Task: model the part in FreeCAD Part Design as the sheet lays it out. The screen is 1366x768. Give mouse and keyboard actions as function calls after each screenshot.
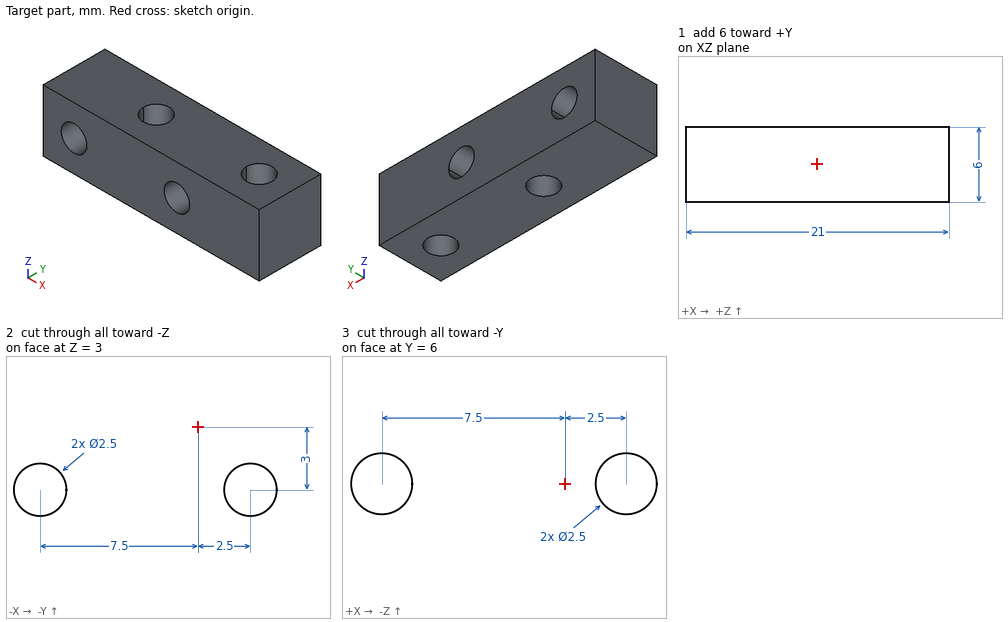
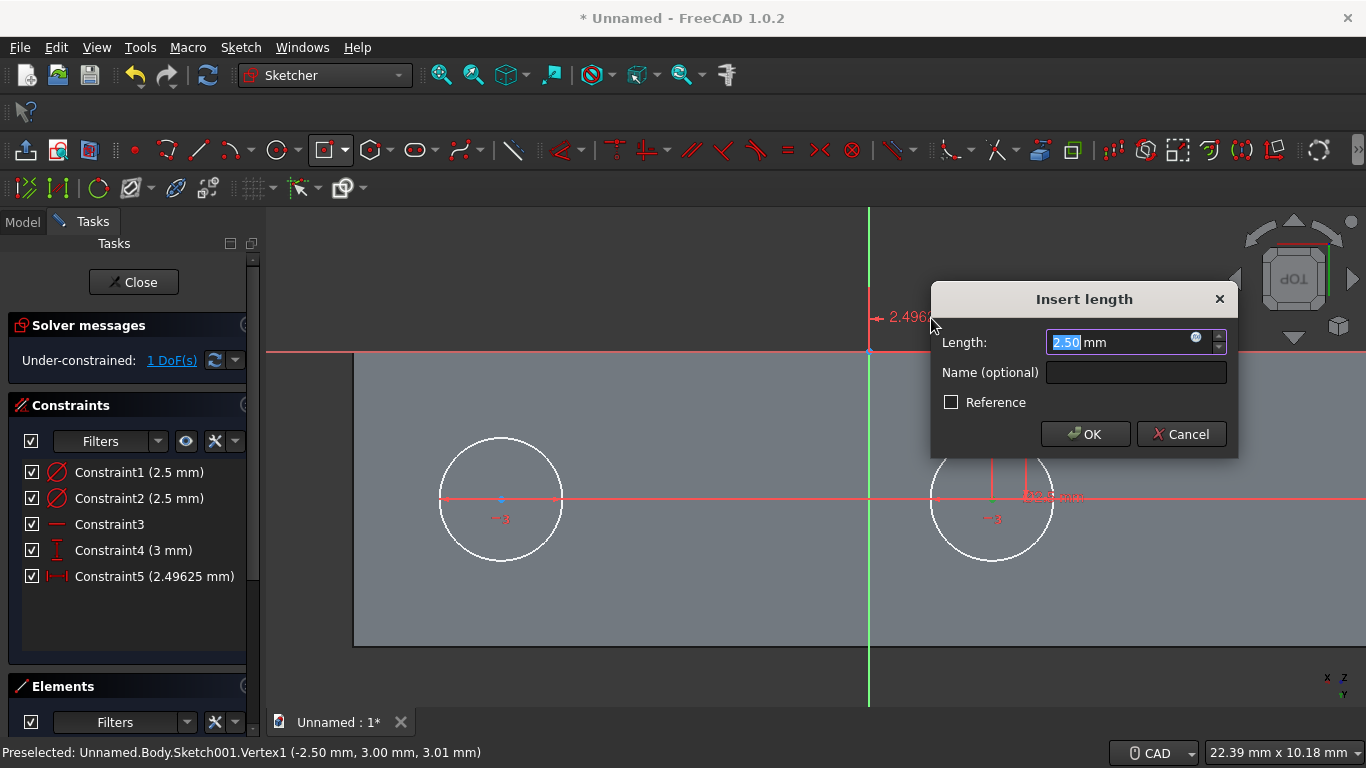
text(2.5)
key(Return)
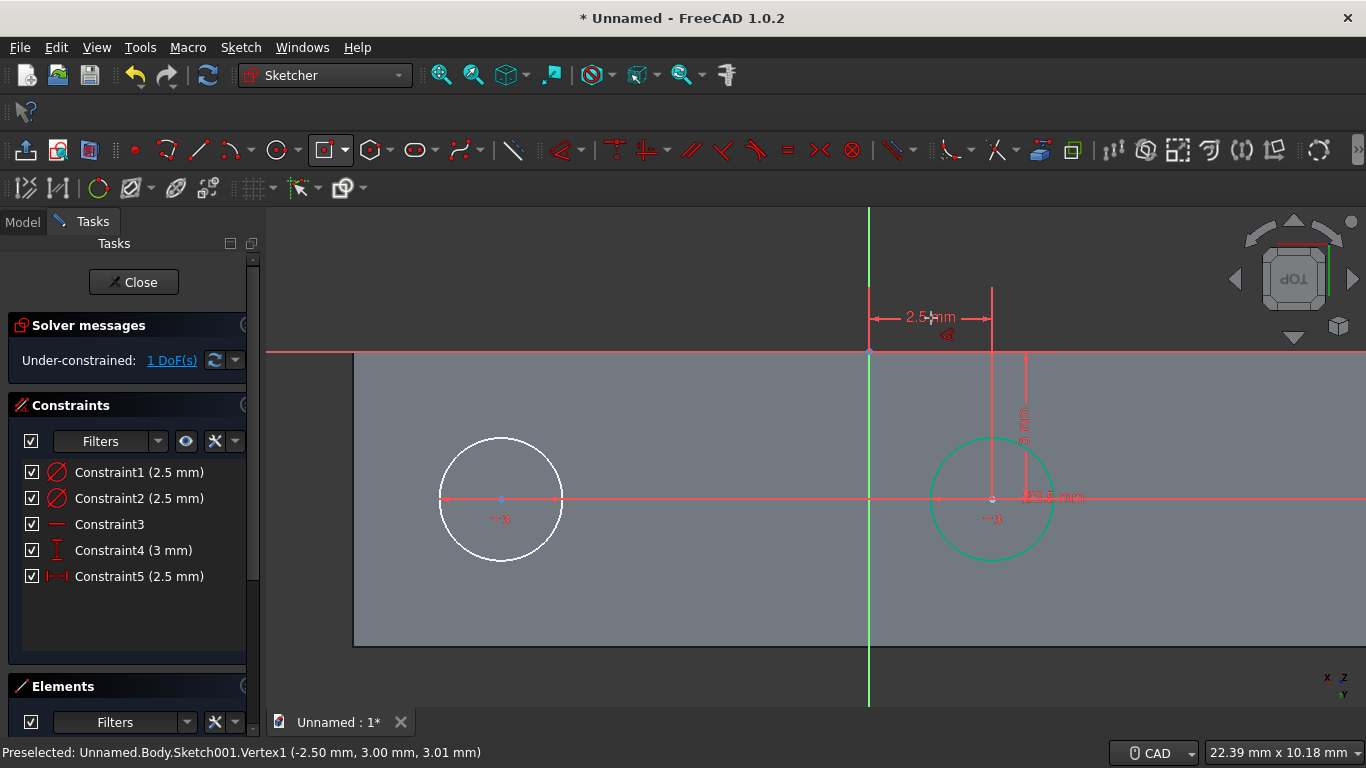
click(501, 499)
click(685, 318)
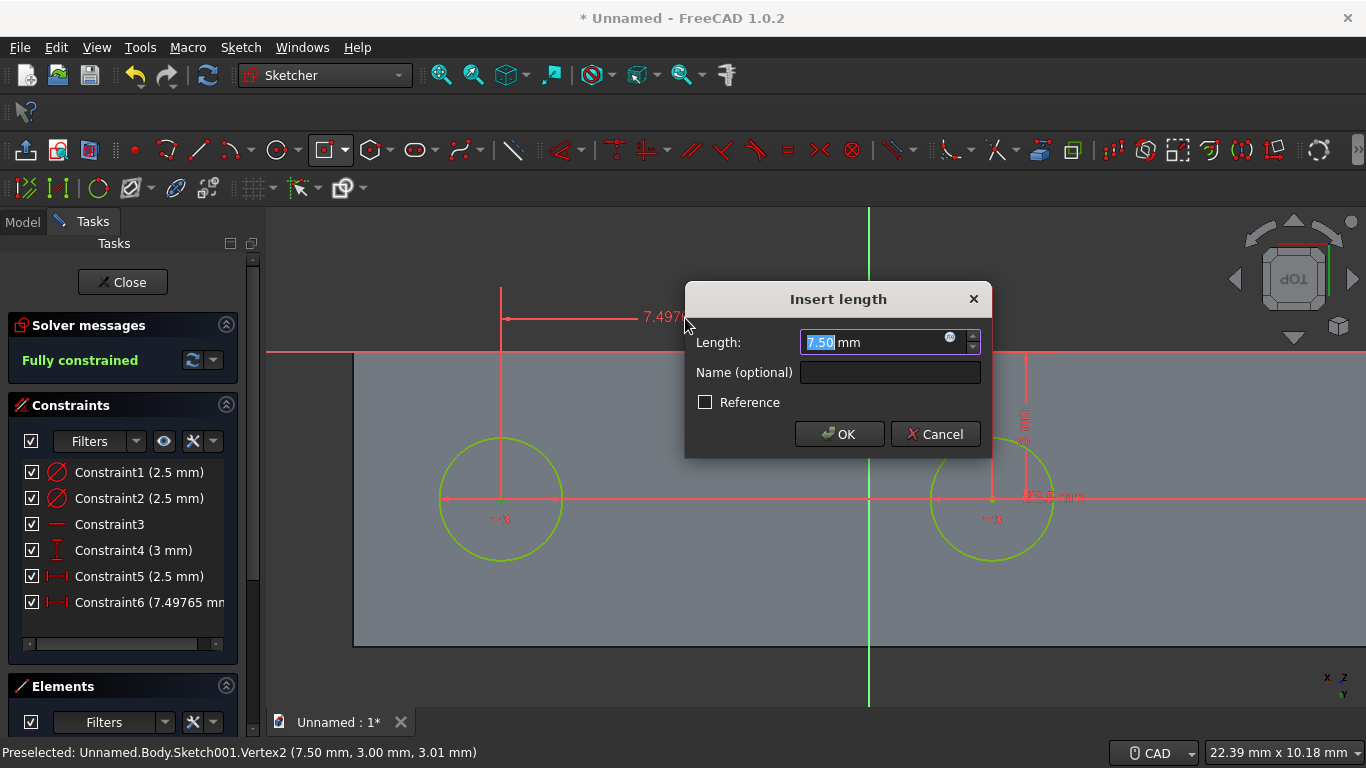
text(7.5)
key(Return)
key(Escape)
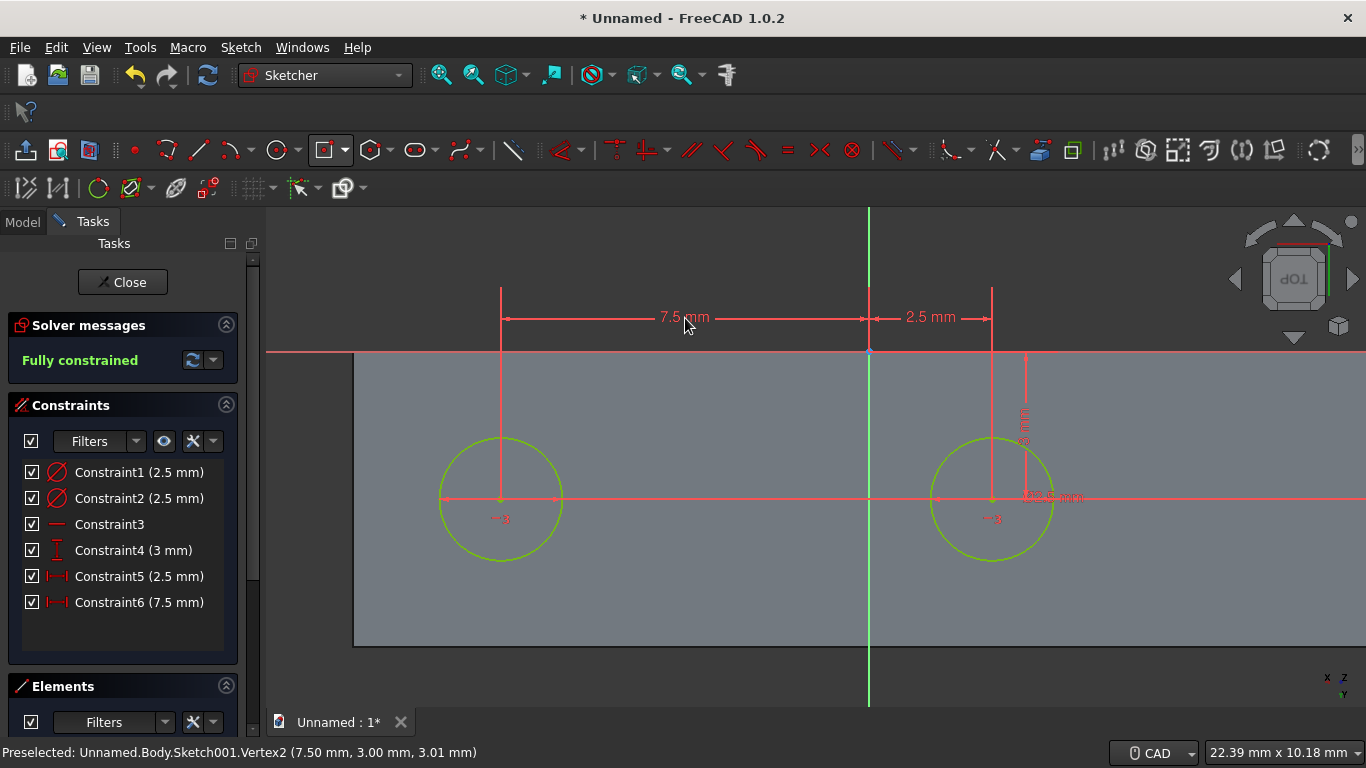
click(123, 282)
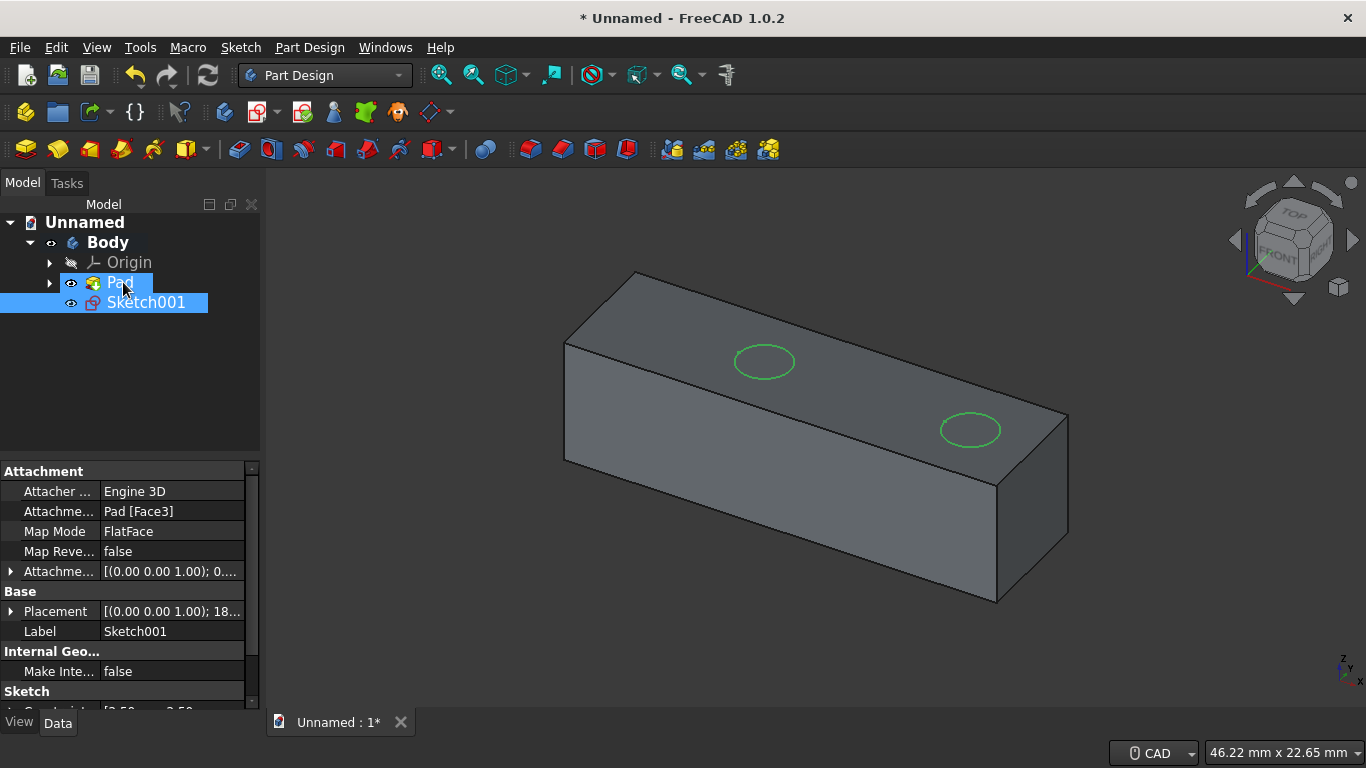
click(240, 150)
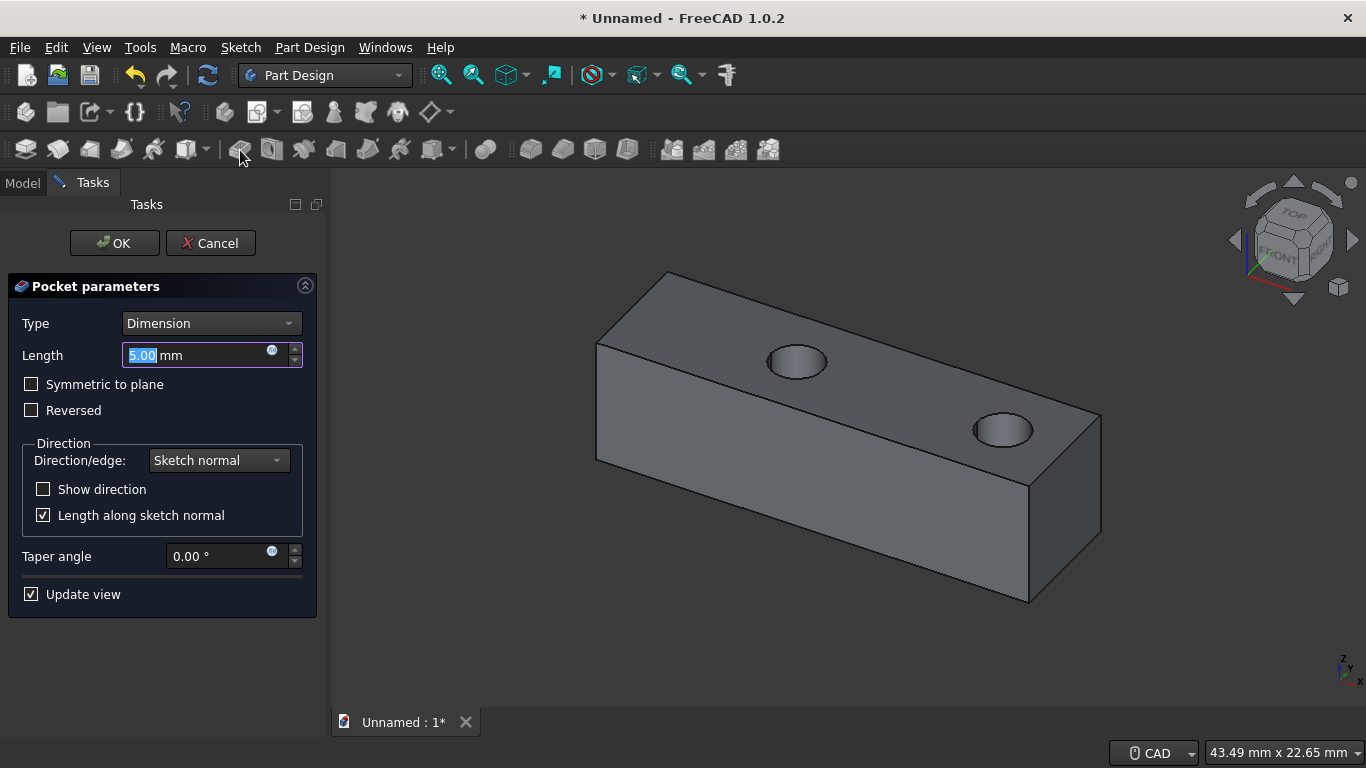
click(212, 324)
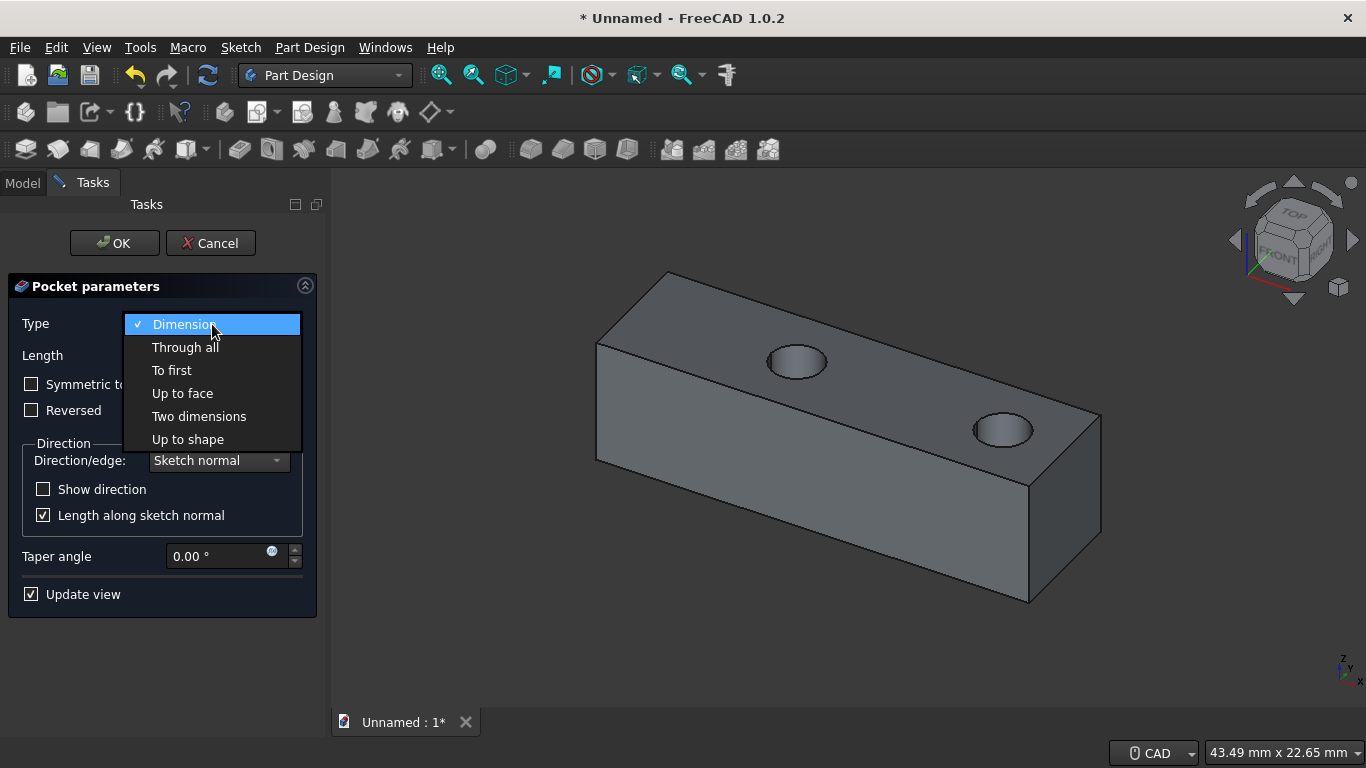
click(212, 348)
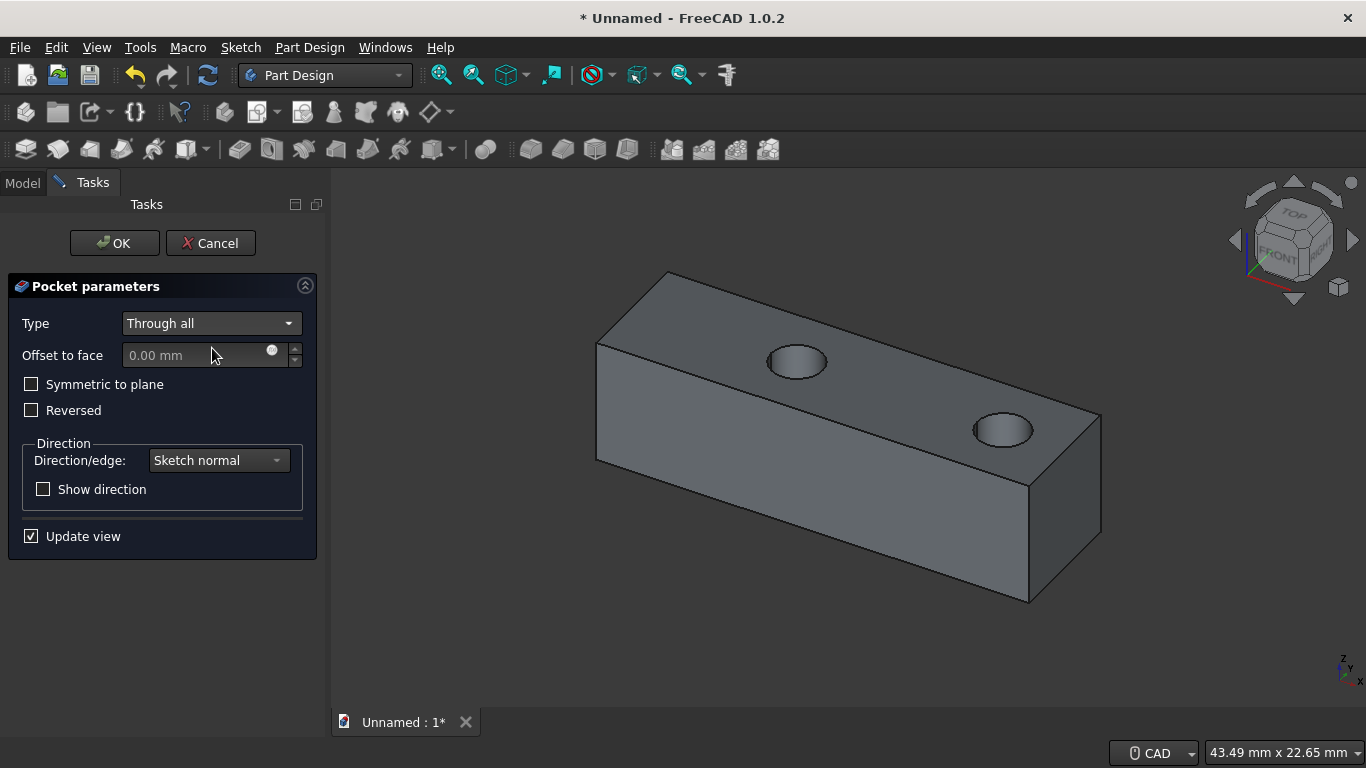
click(115, 243)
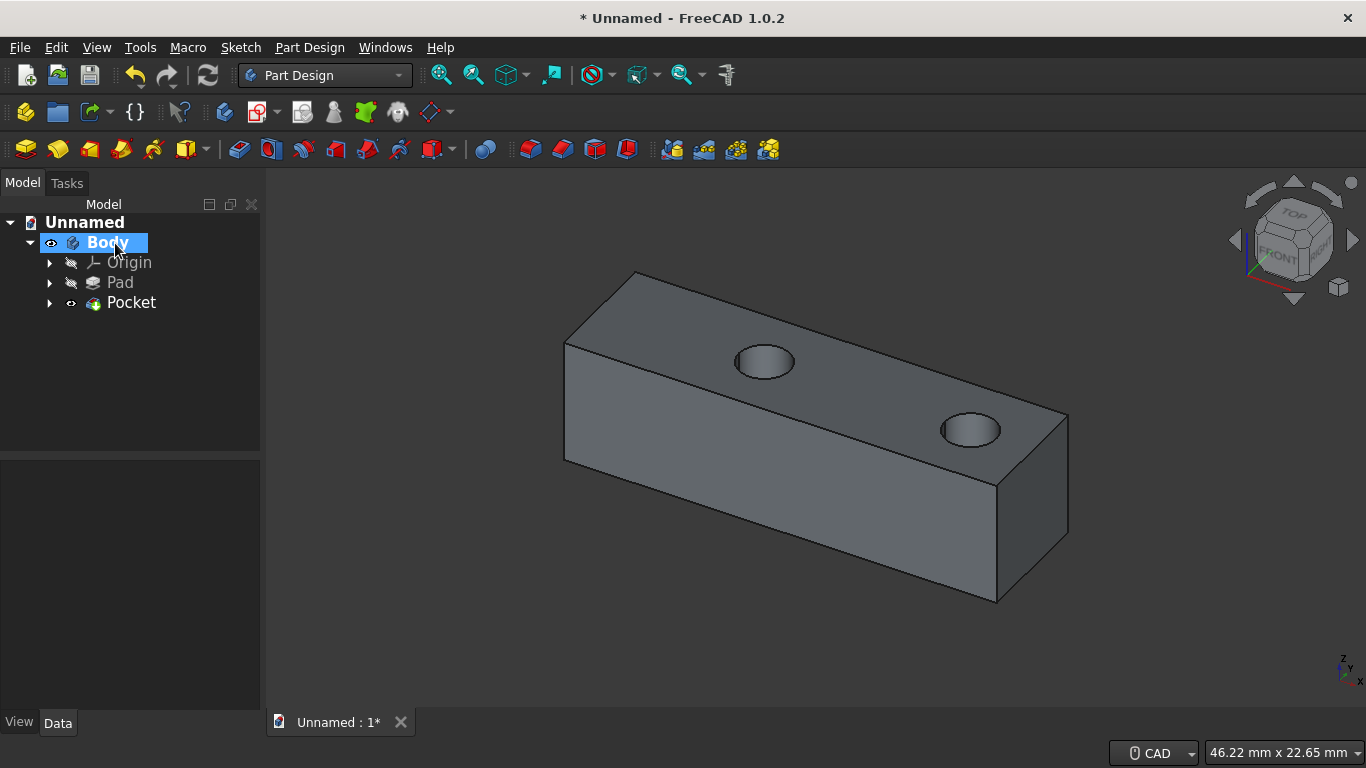
key(4)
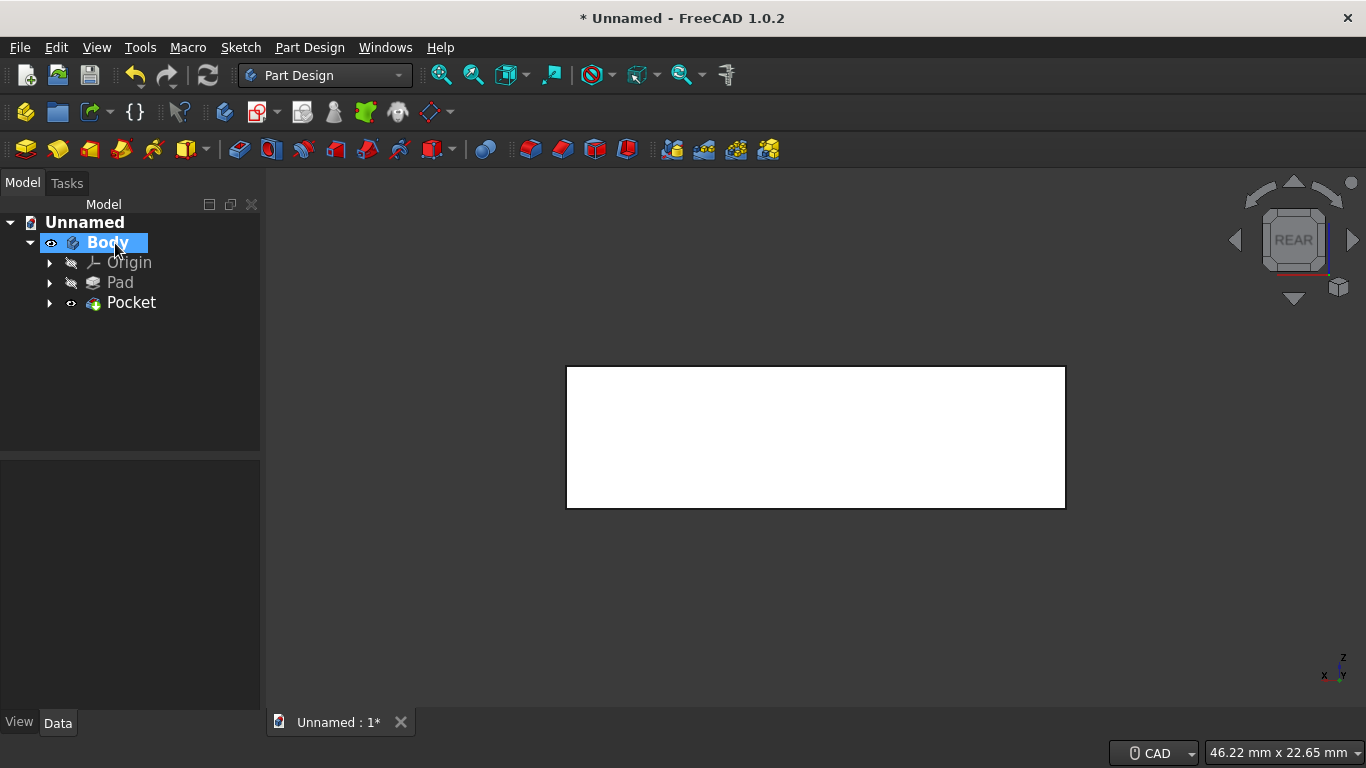
click(673, 437)